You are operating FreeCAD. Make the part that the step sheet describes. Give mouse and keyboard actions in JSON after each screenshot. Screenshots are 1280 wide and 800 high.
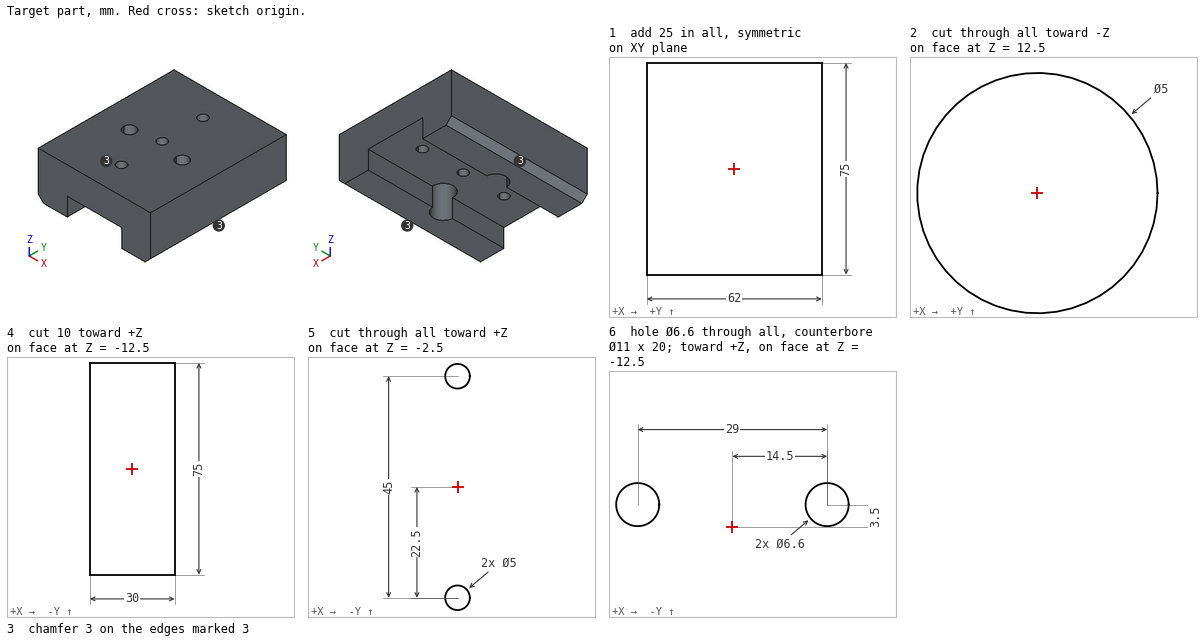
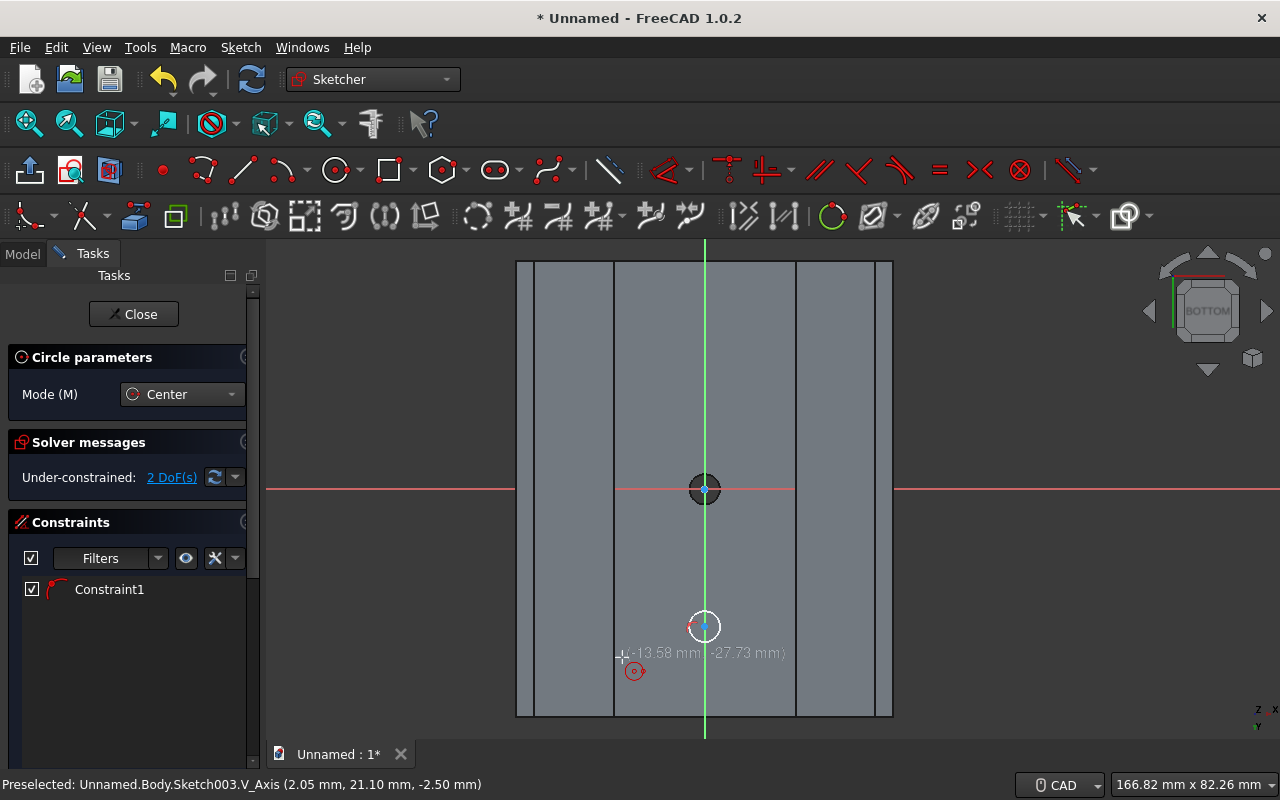
{"action": "scroll", "coordinate": [705, 353], "scroll_direction": "up", "scroll_amount": 3}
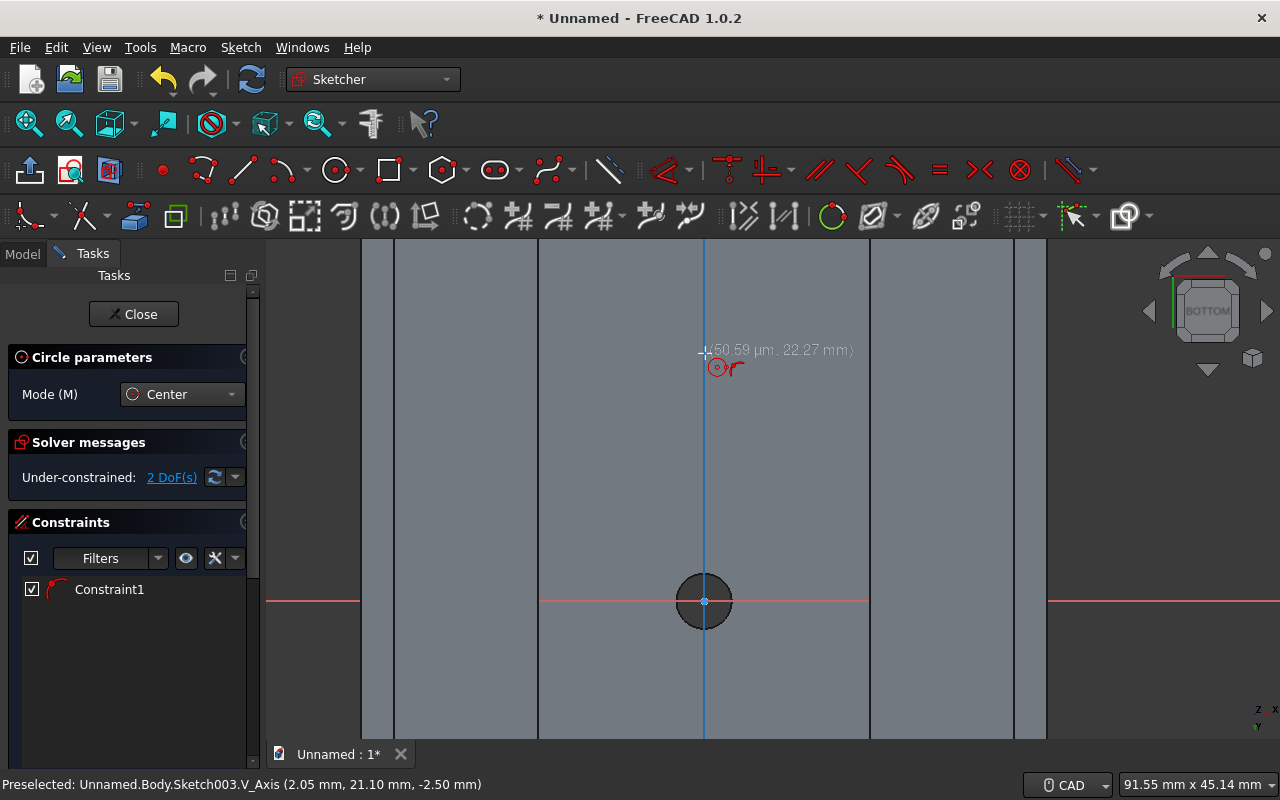
{"action": "left_click", "coordinate": [704, 352]}
{"action": "left_click", "coordinate": [724, 332]}
{"action": "key", "text": "Escape"}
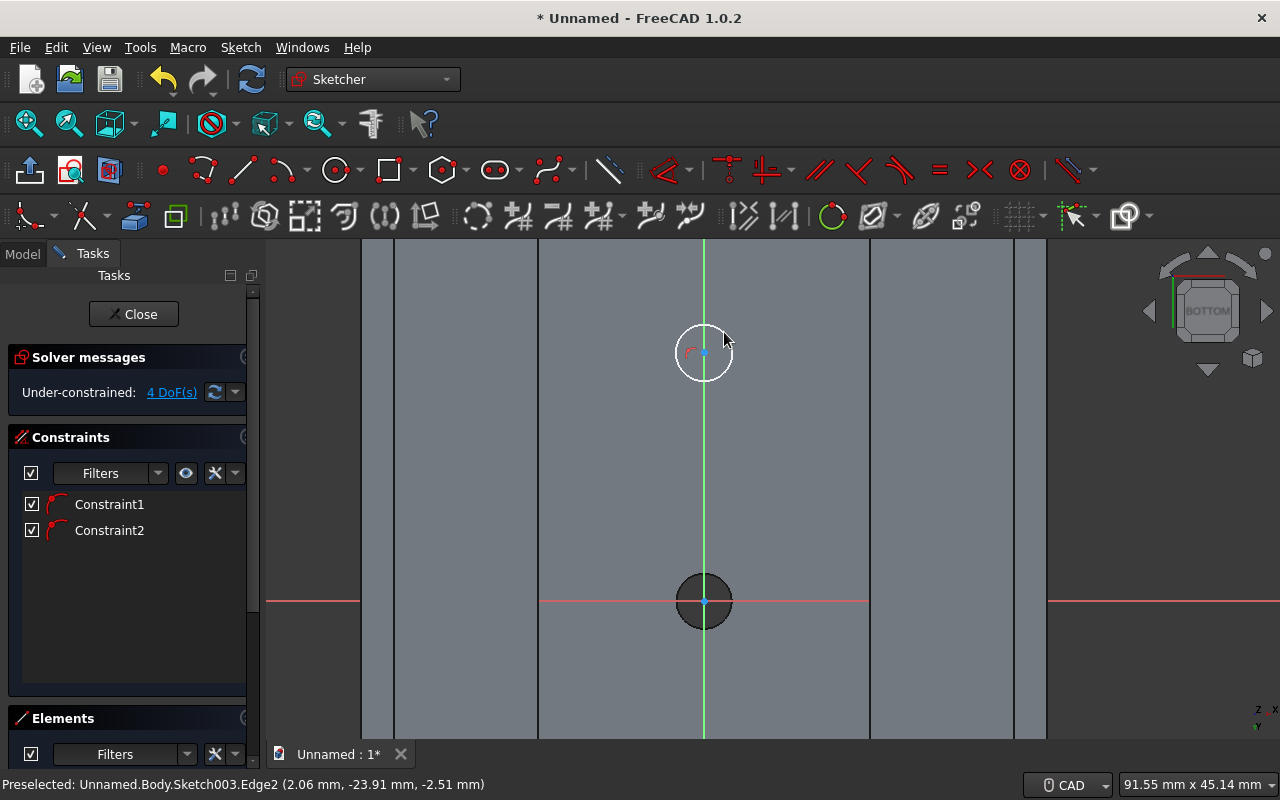
{"action": "scroll", "coordinate": [705, 352], "scroll_direction": "down", "scroll_amount": 3}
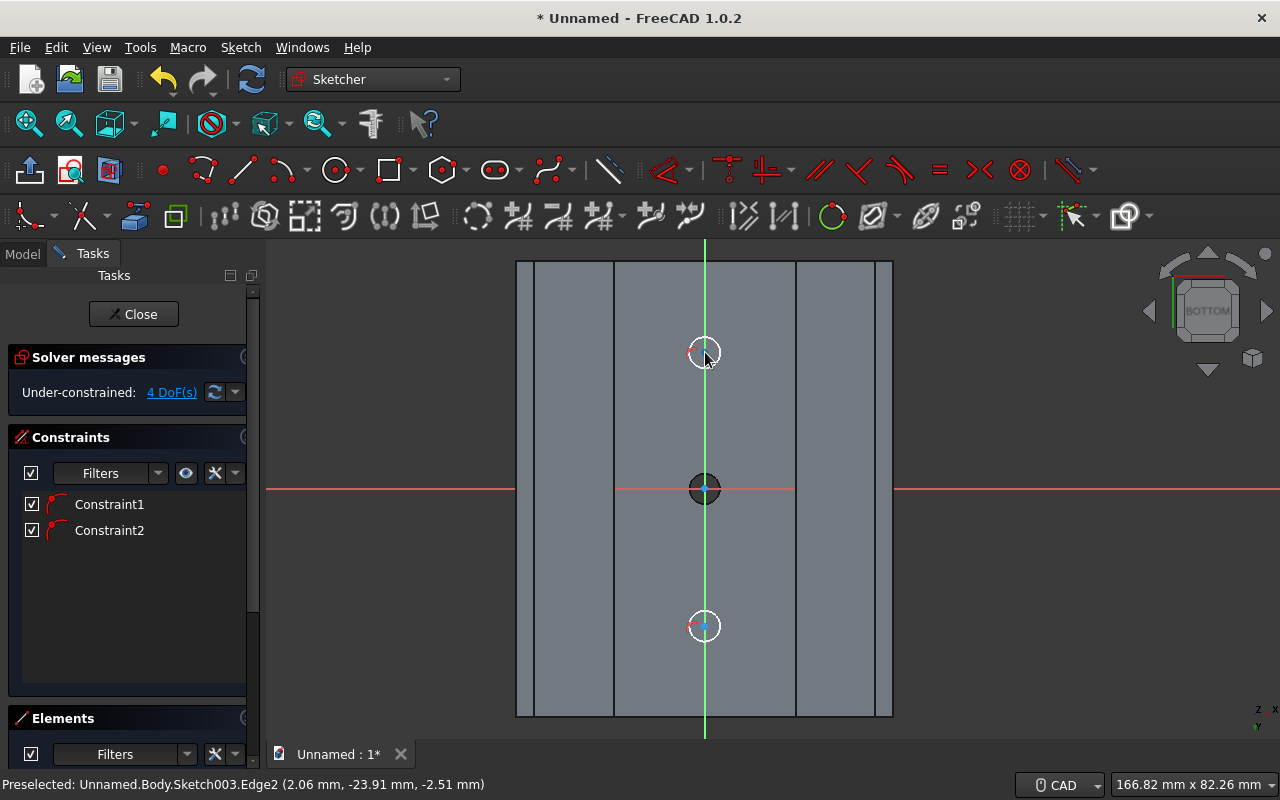
{"action": "scroll", "coordinate": [716, 615], "scroll_direction": "up", "scroll_amount": 2}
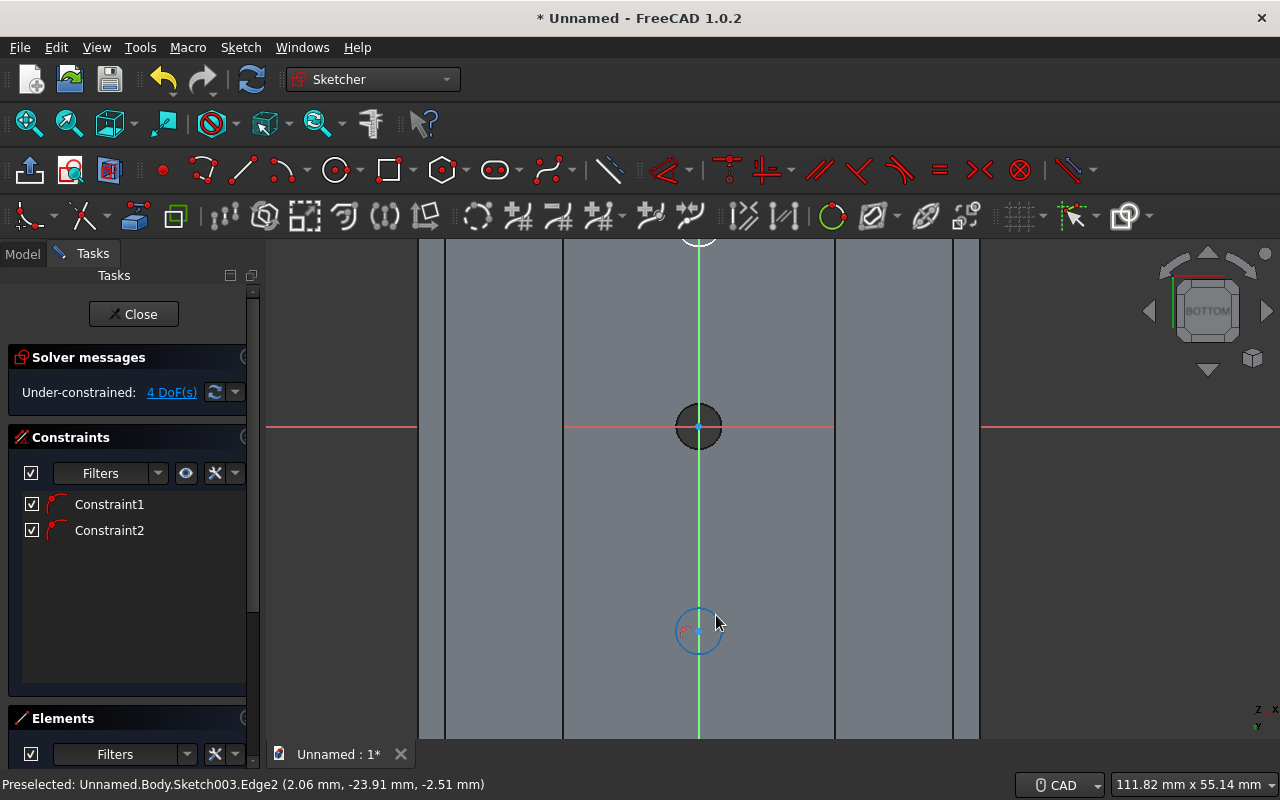
{"action": "left_click", "coordinate": [715, 615]}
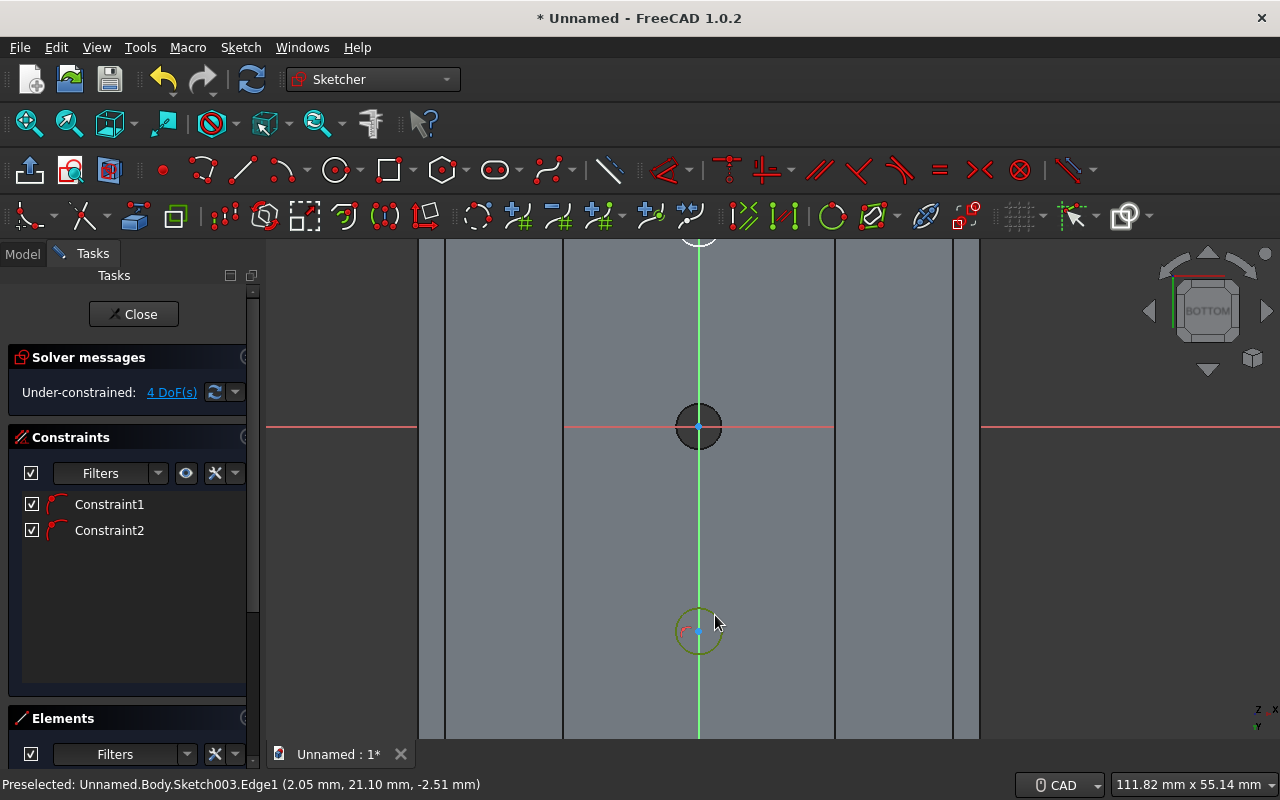
{"action": "scroll", "coordinate": [716, 616], "scroll_direction": "down", "scroll_amount": 2}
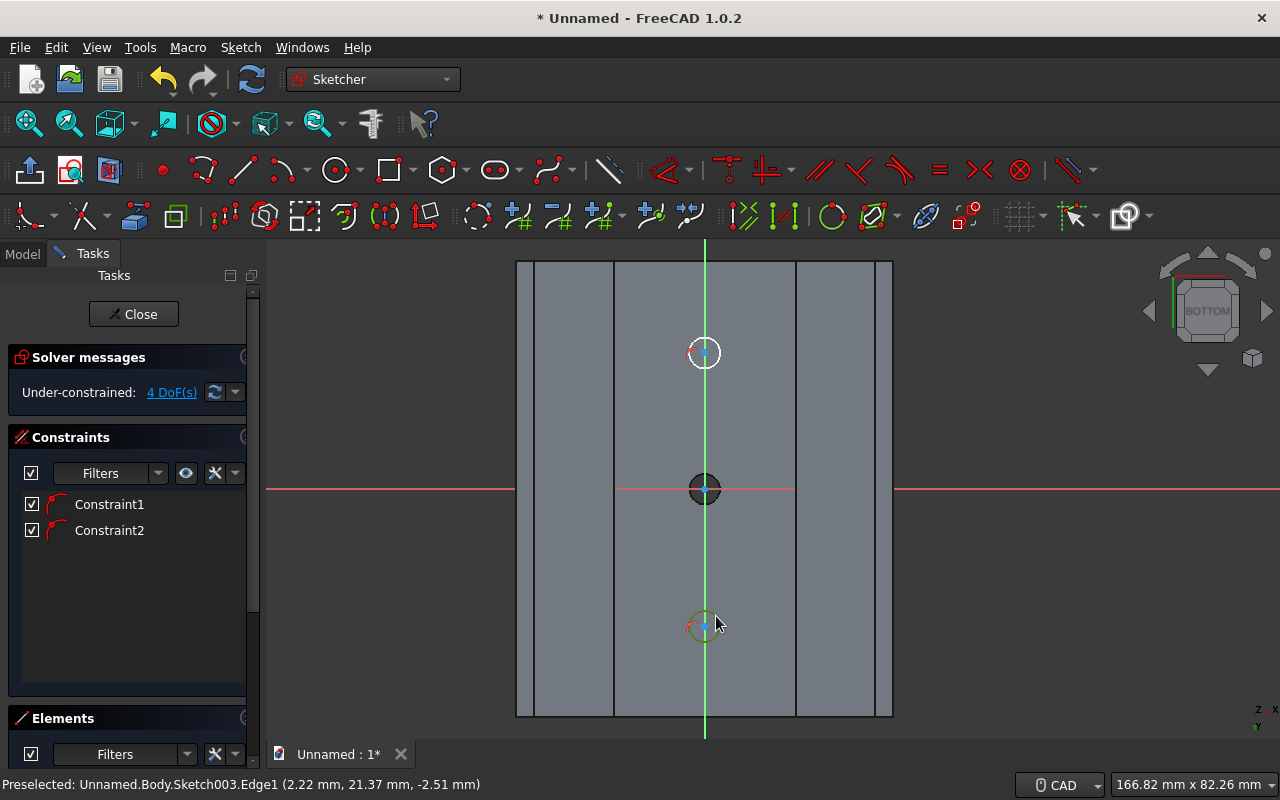
{"action": "scroll", "coordinate": [716, 342], "scroll_direction": "up", "scroll_amount": 2}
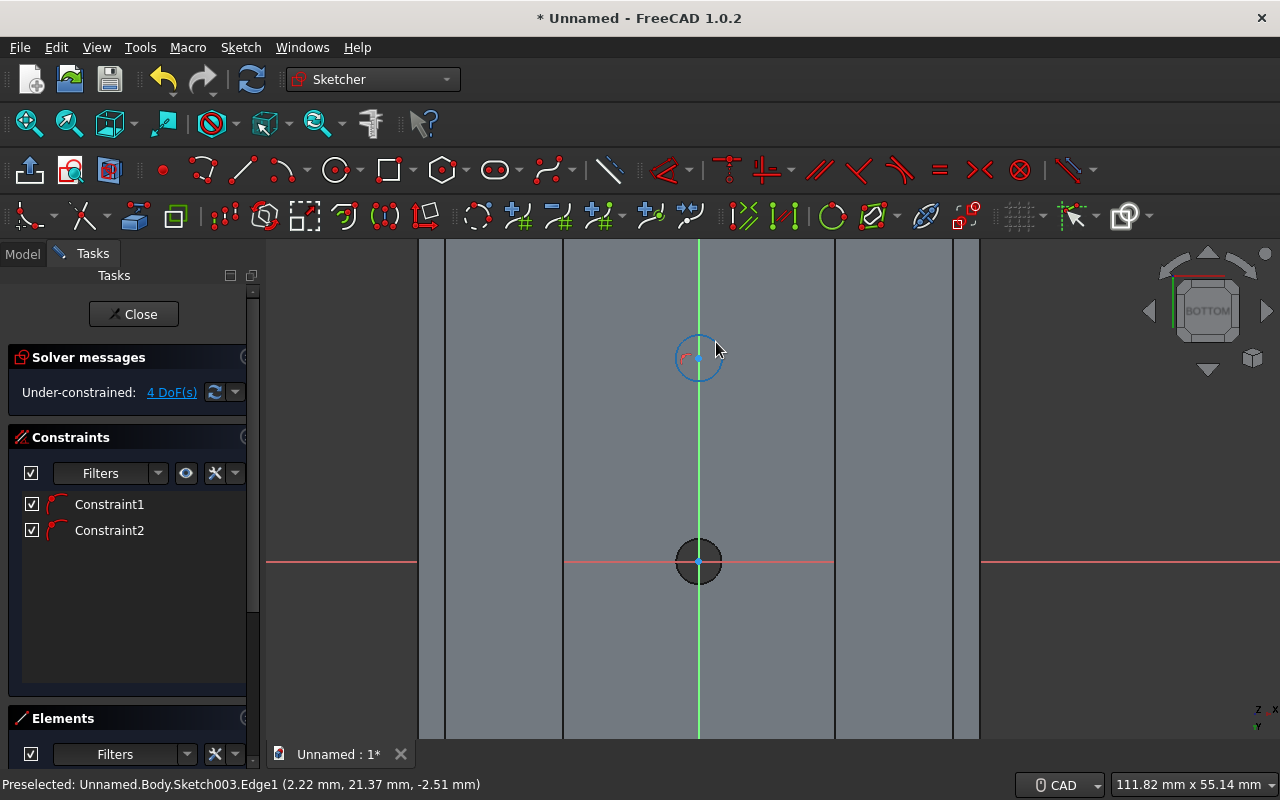
{"action": "left_click", "coordinate": [715, 342]}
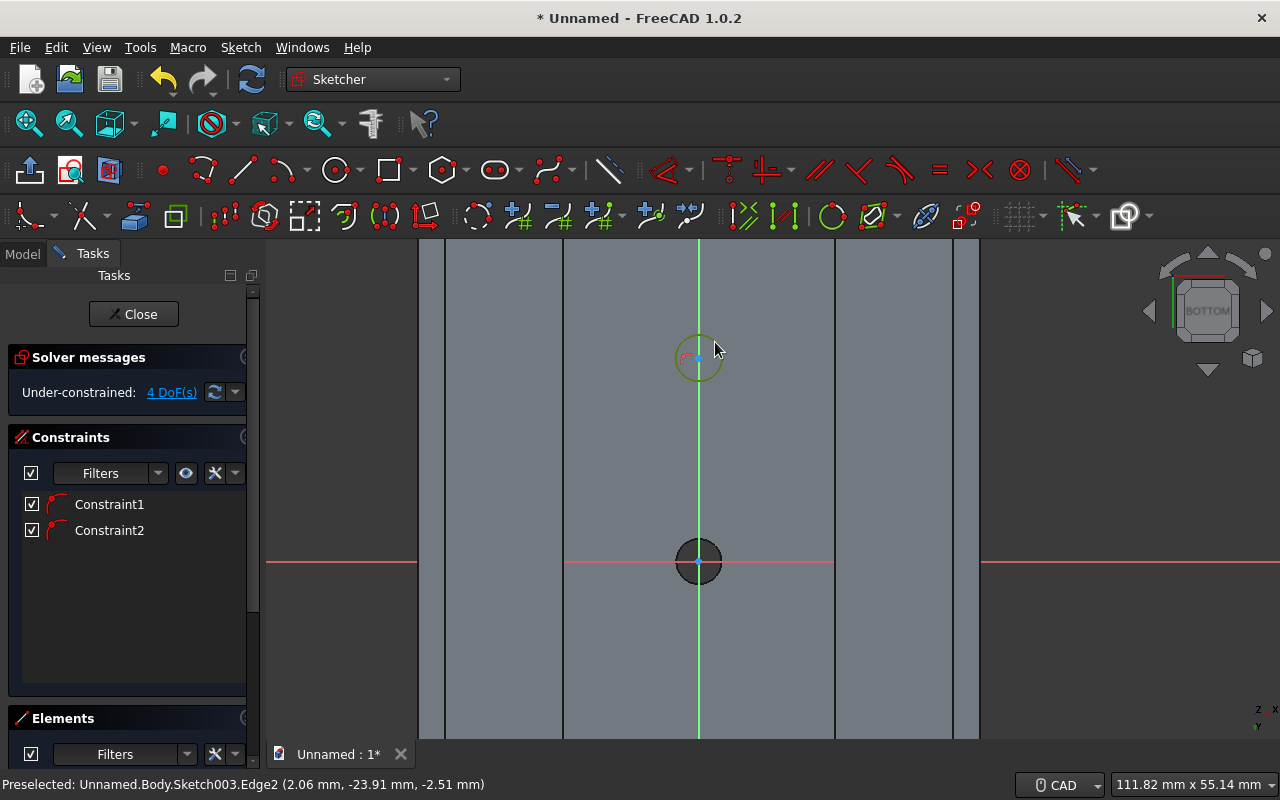
{"action": "key", "text": "e"}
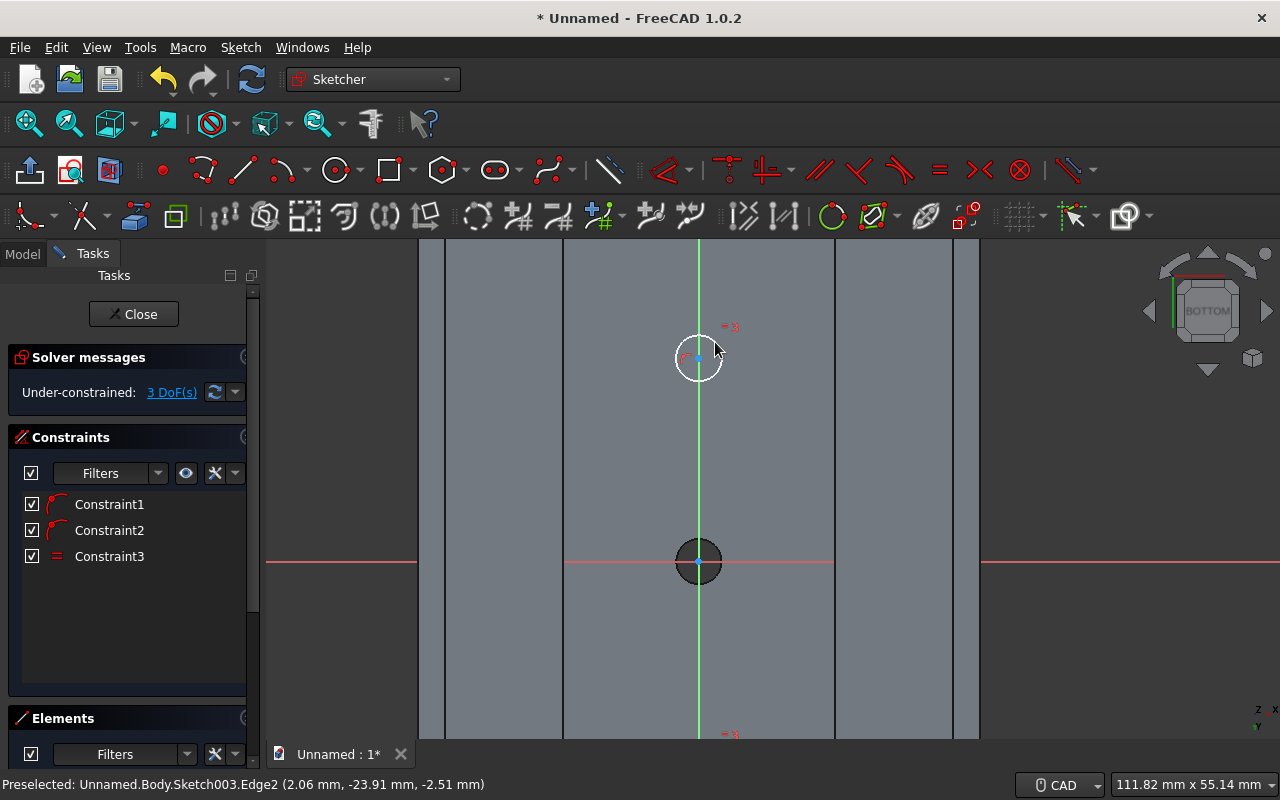
{"action": "left_click", "coordinate": [664, 170]}